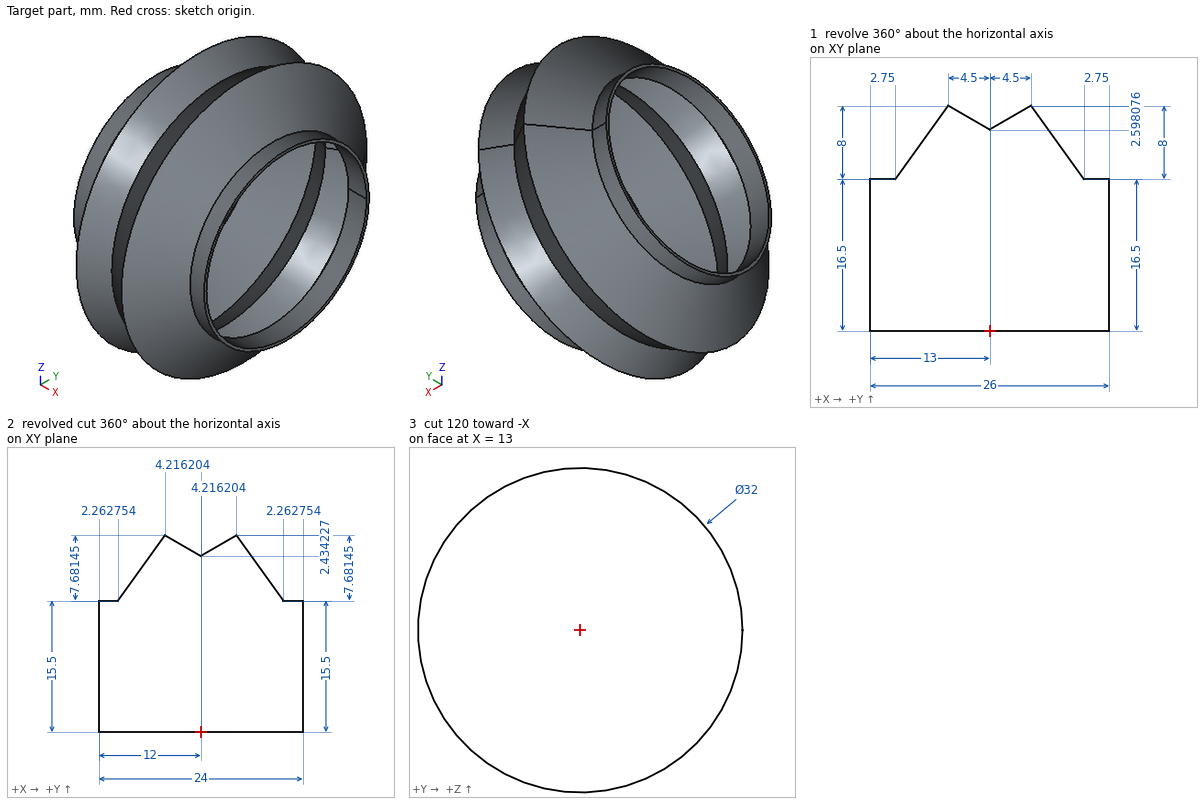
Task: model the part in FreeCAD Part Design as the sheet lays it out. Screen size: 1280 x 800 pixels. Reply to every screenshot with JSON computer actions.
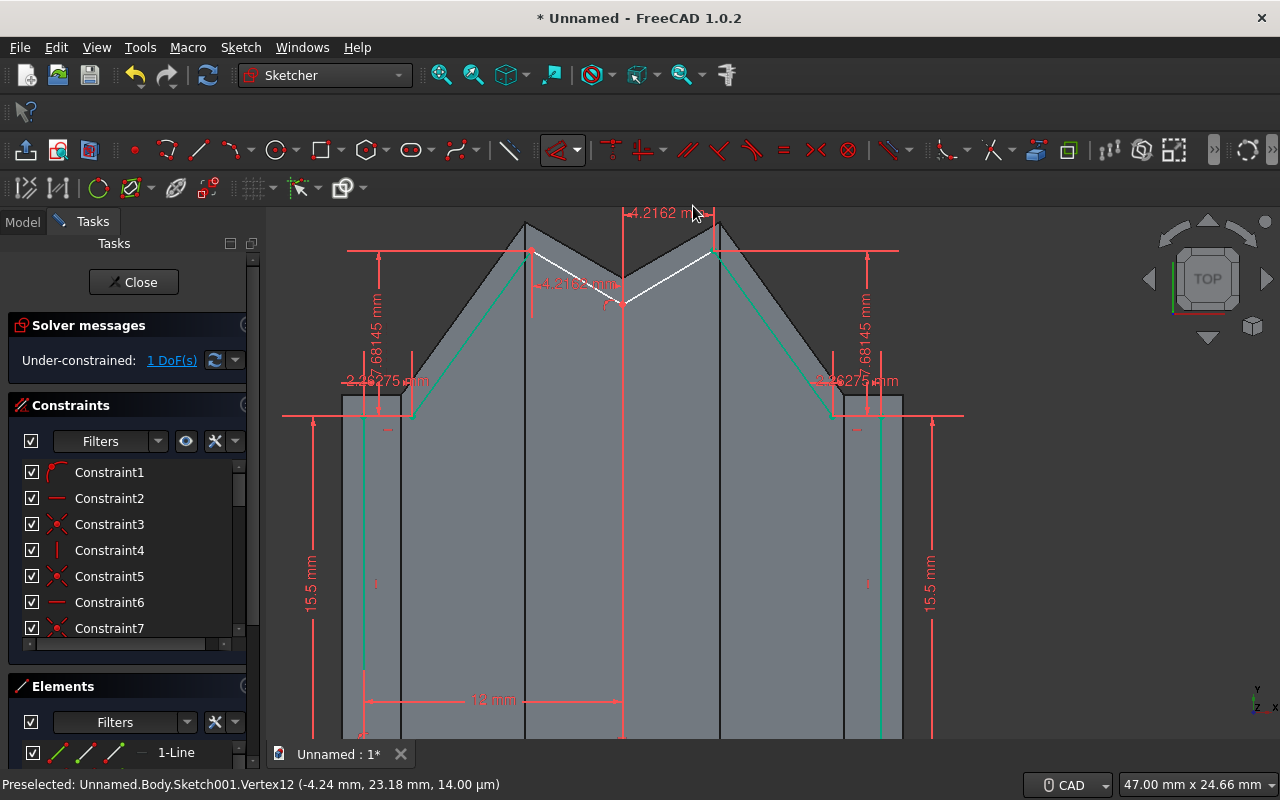
{"action": "left_click", "coordinate": [686, 267]}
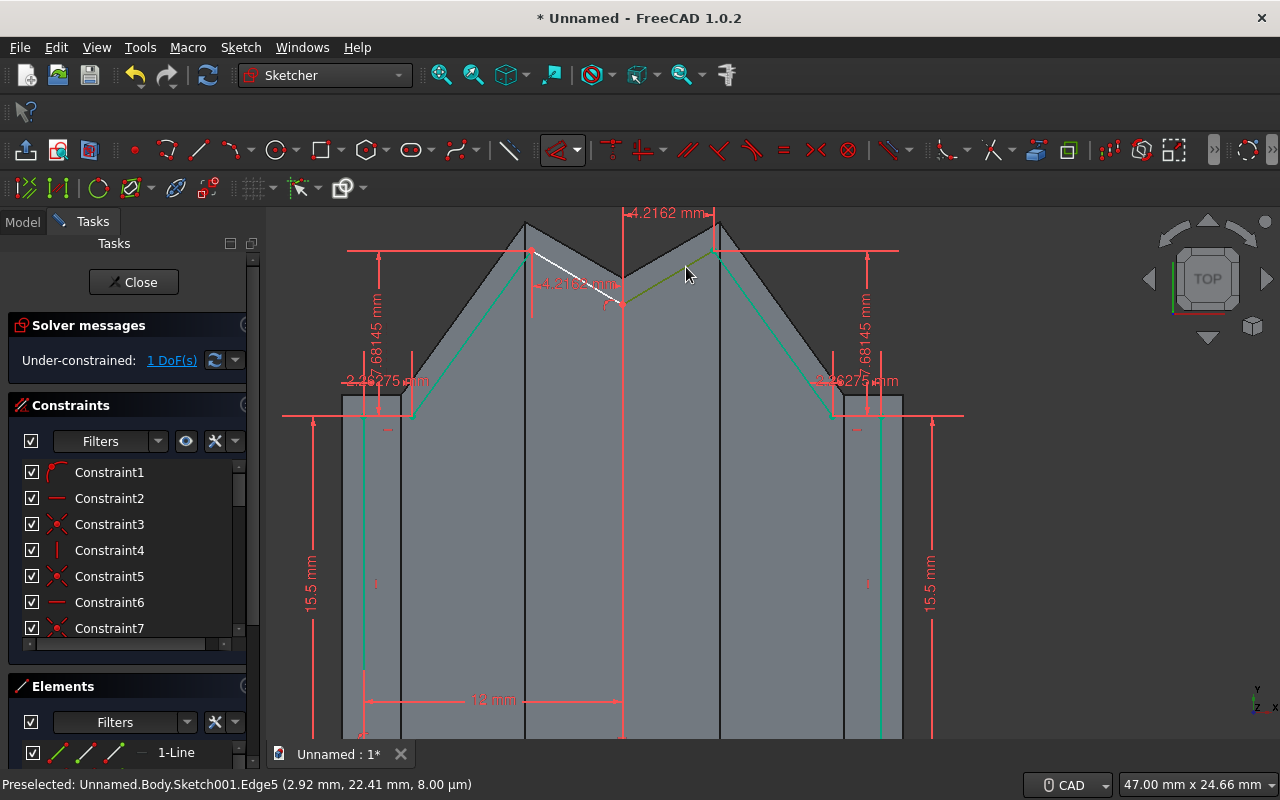
{"action": "key", "text": "i"}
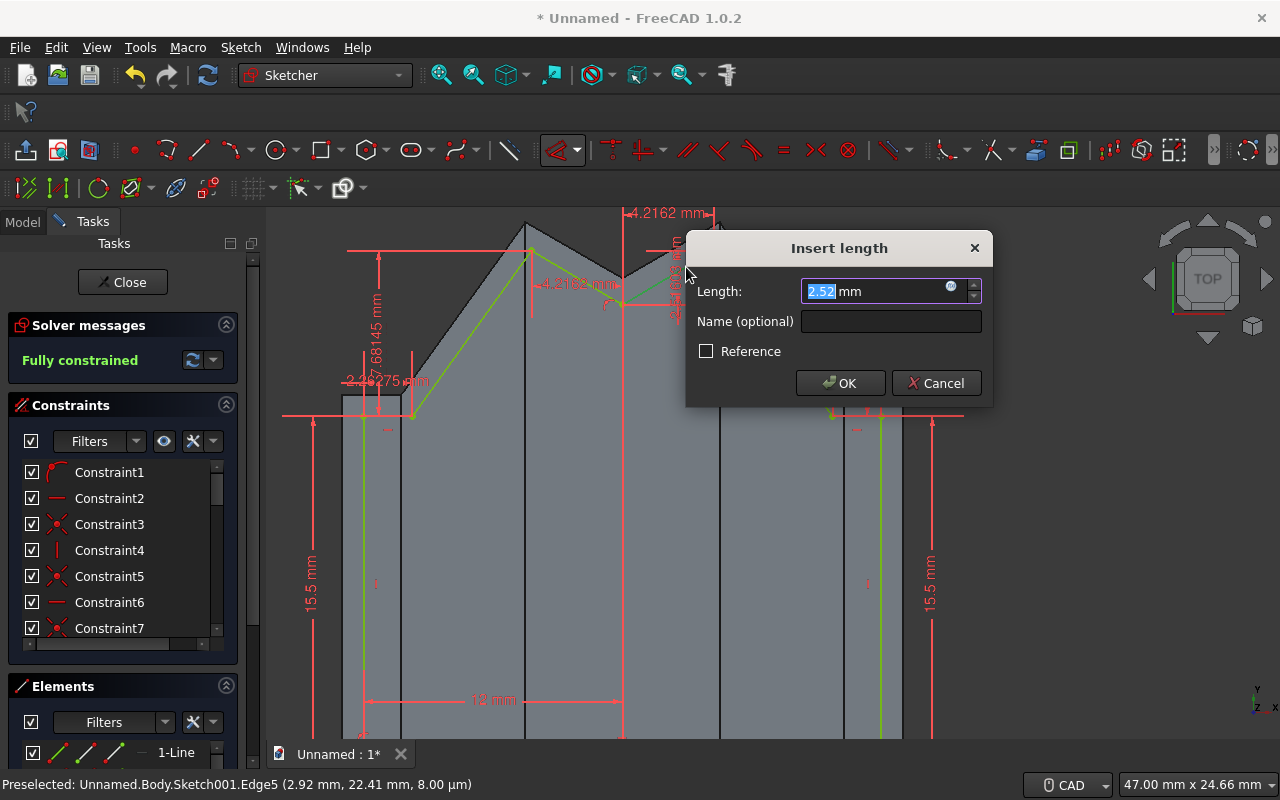
{"action": "type", "text": "2.434227"}
{"action": "key", "text": "Return"}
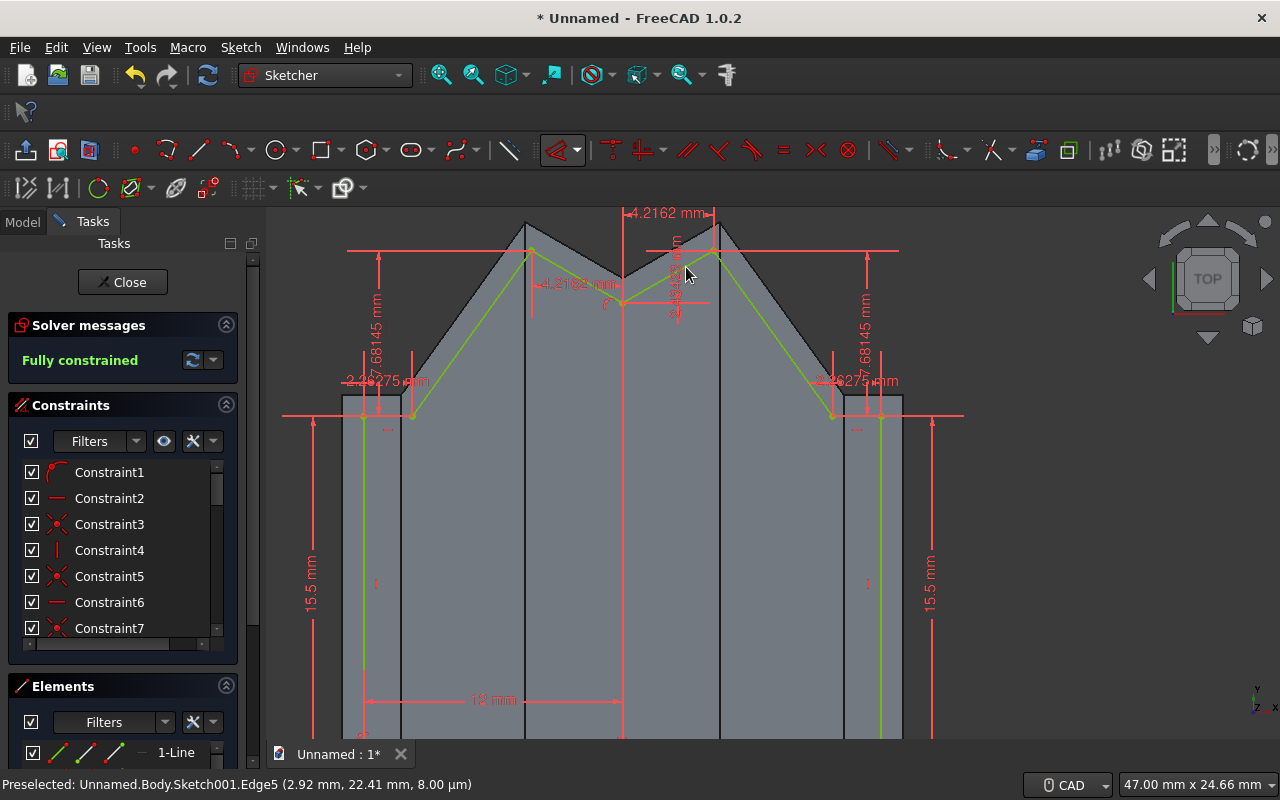
{"action": "left_click", "coordinate": [123, 282]}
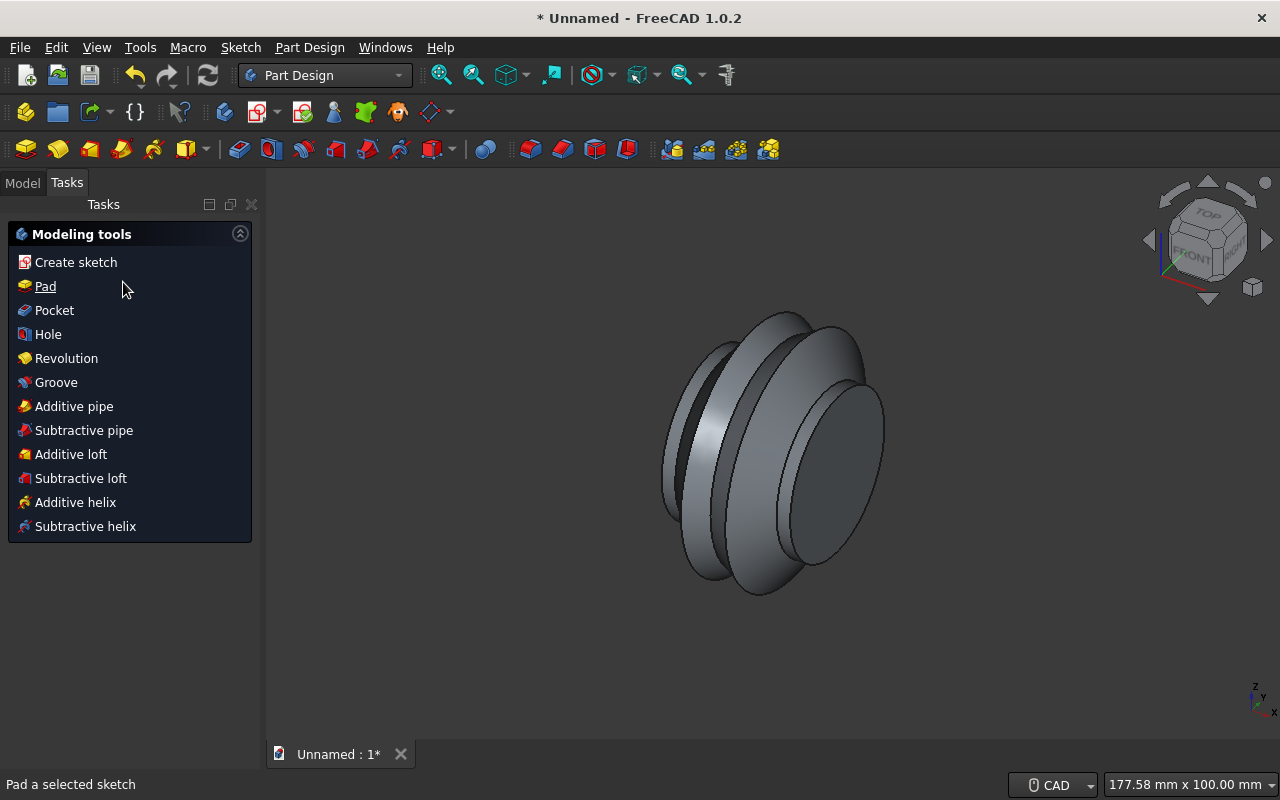
{"action": "left_click", "coordinate": [304, 150]}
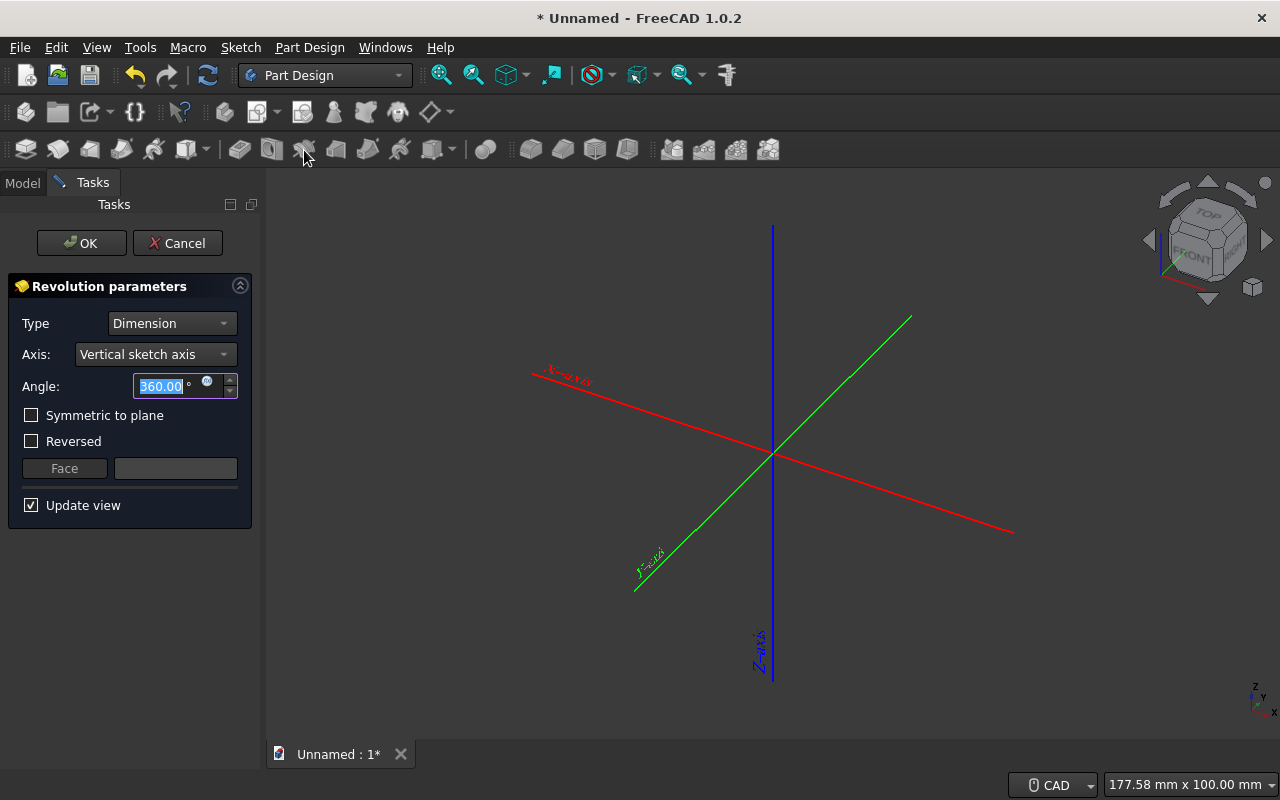
{"action": "left_click", "coordinate": [156, 354]}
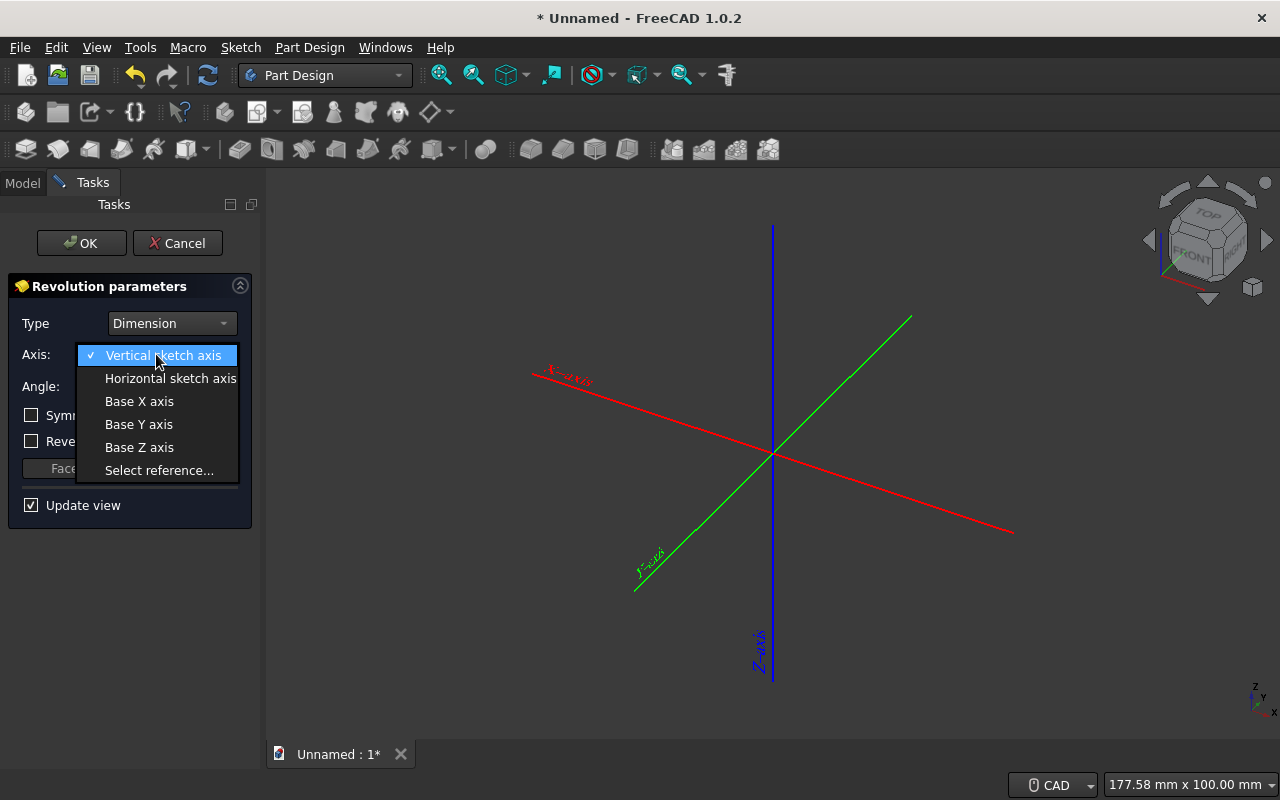
{"action": "left_click", "coordinate": [156, 378]}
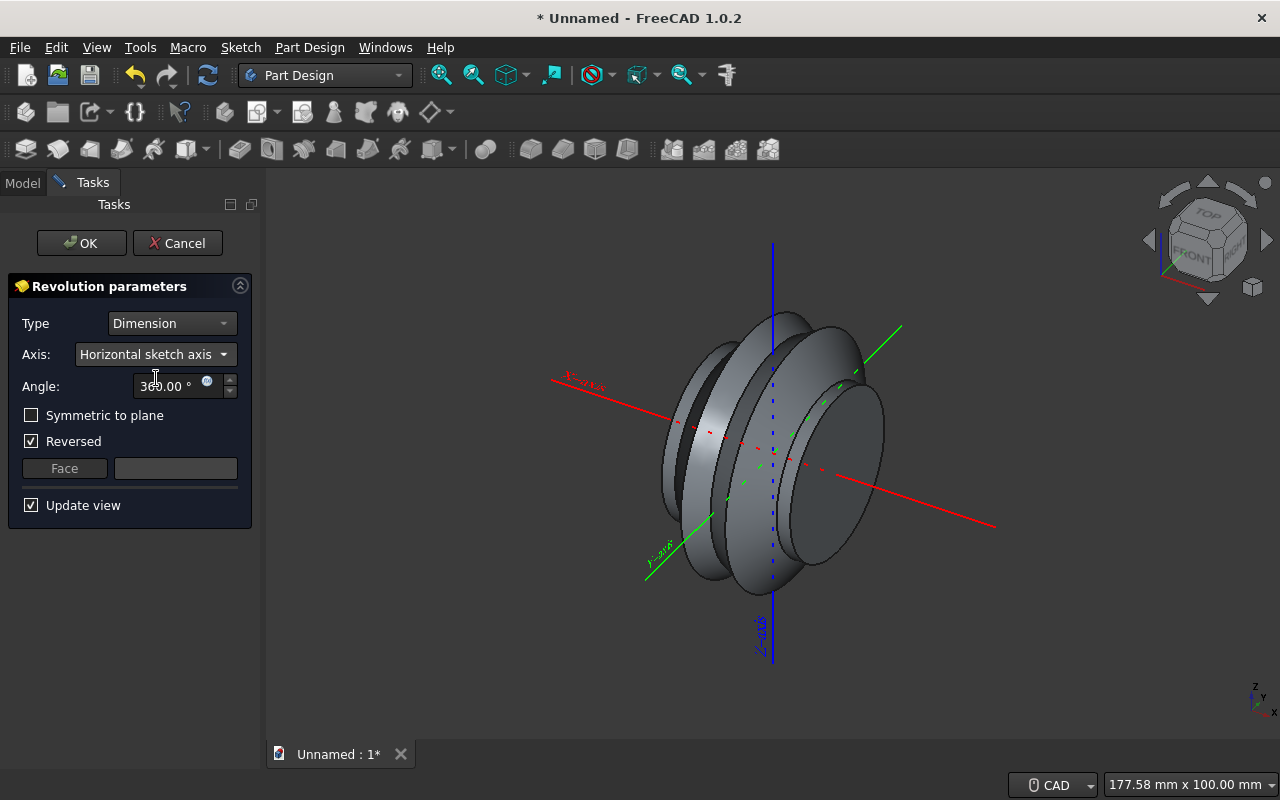
{"action": "left_click", "coordinate": [82, 243]}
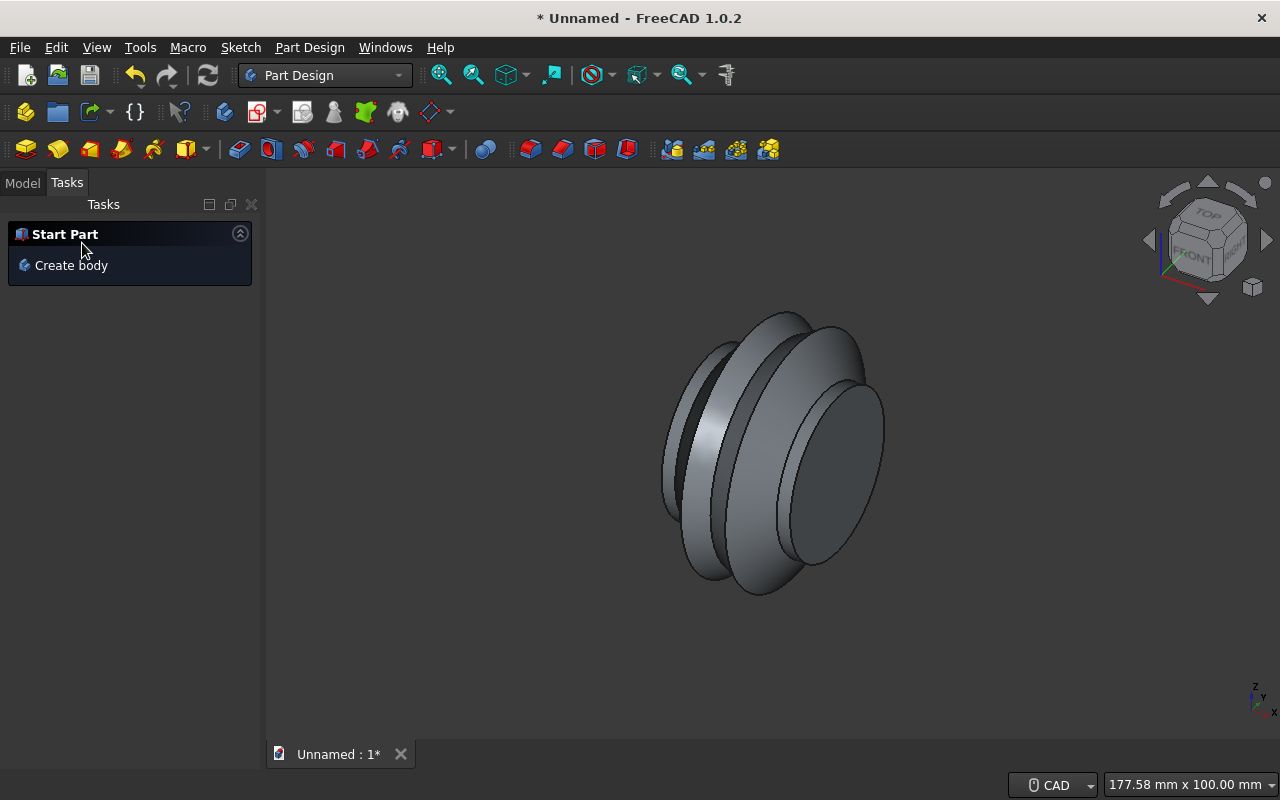
{"action": "left_click", "coordinate": [837, 474]}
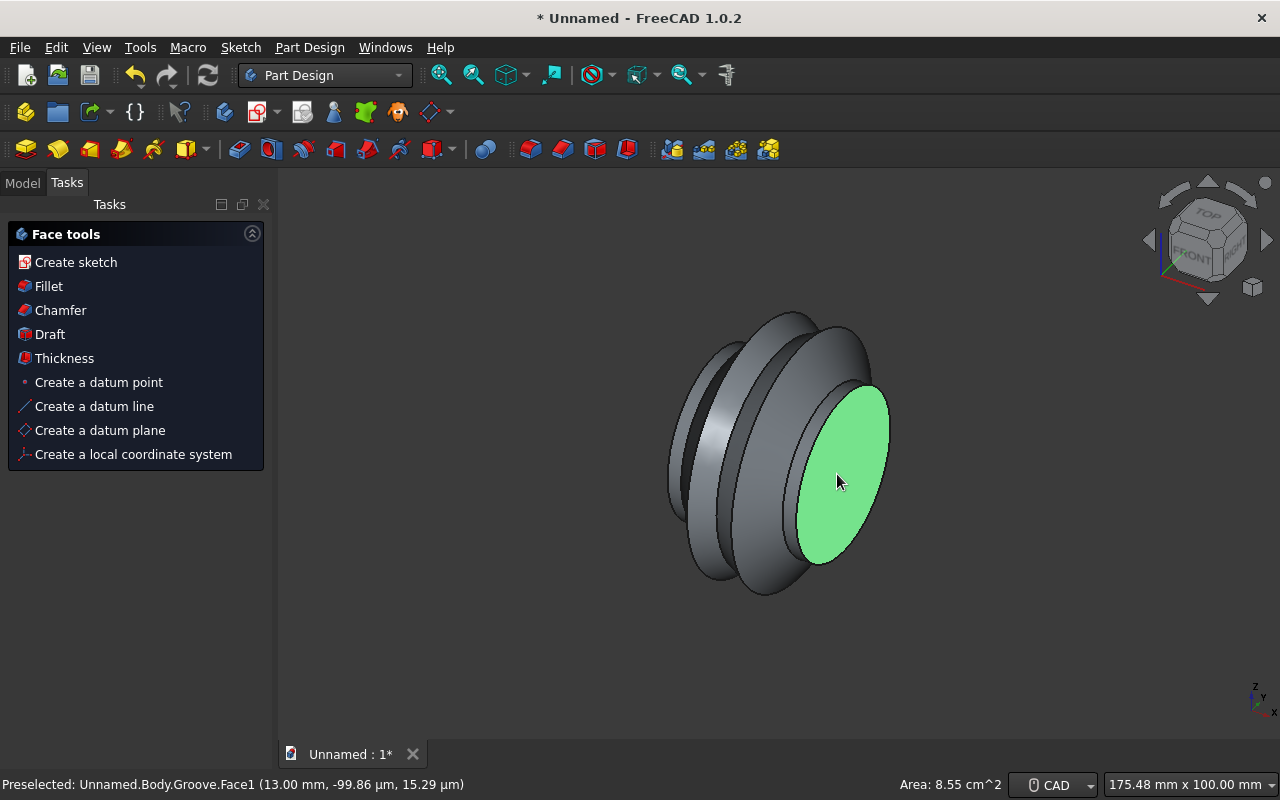
{"action": "left_click", "coordinate": [258, 112]}